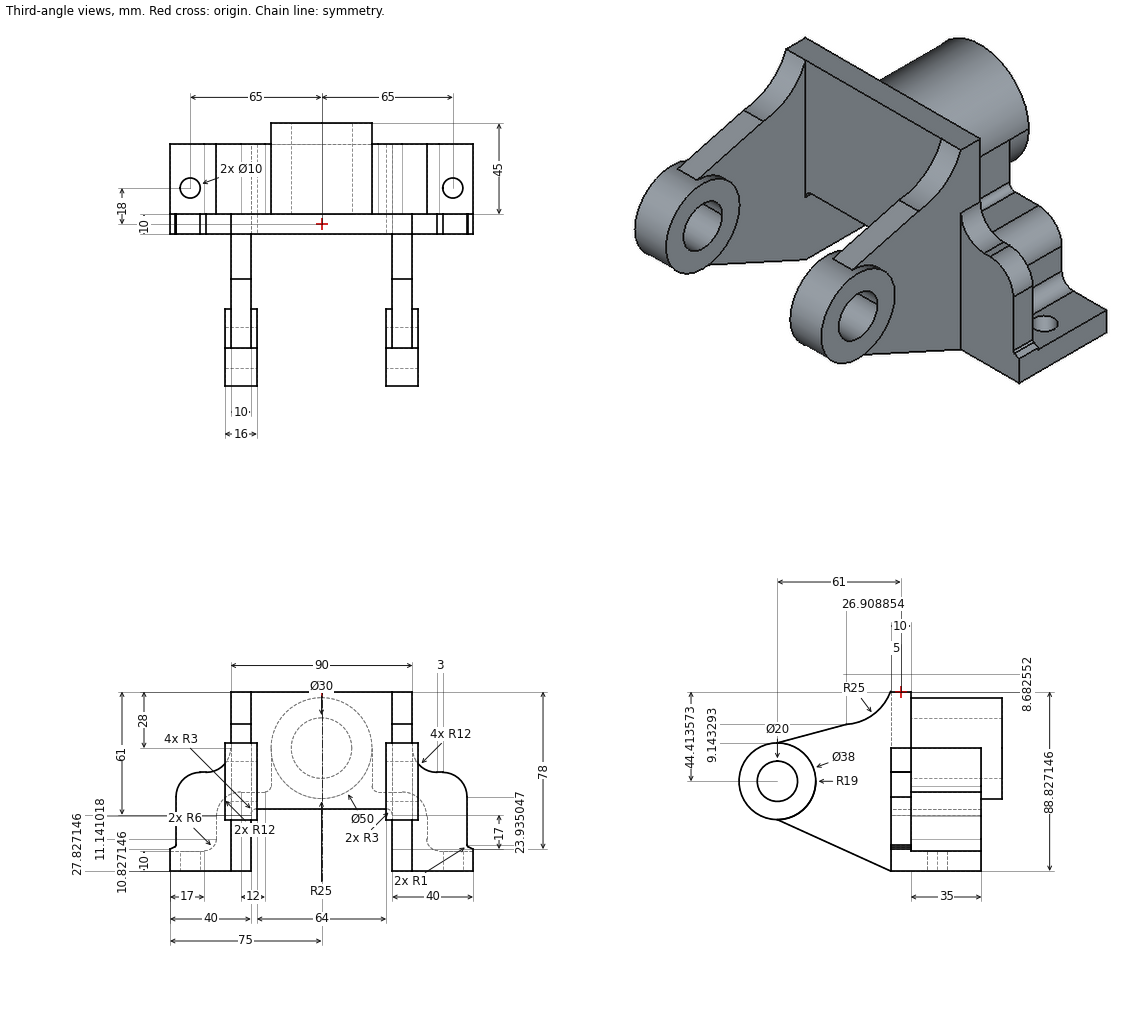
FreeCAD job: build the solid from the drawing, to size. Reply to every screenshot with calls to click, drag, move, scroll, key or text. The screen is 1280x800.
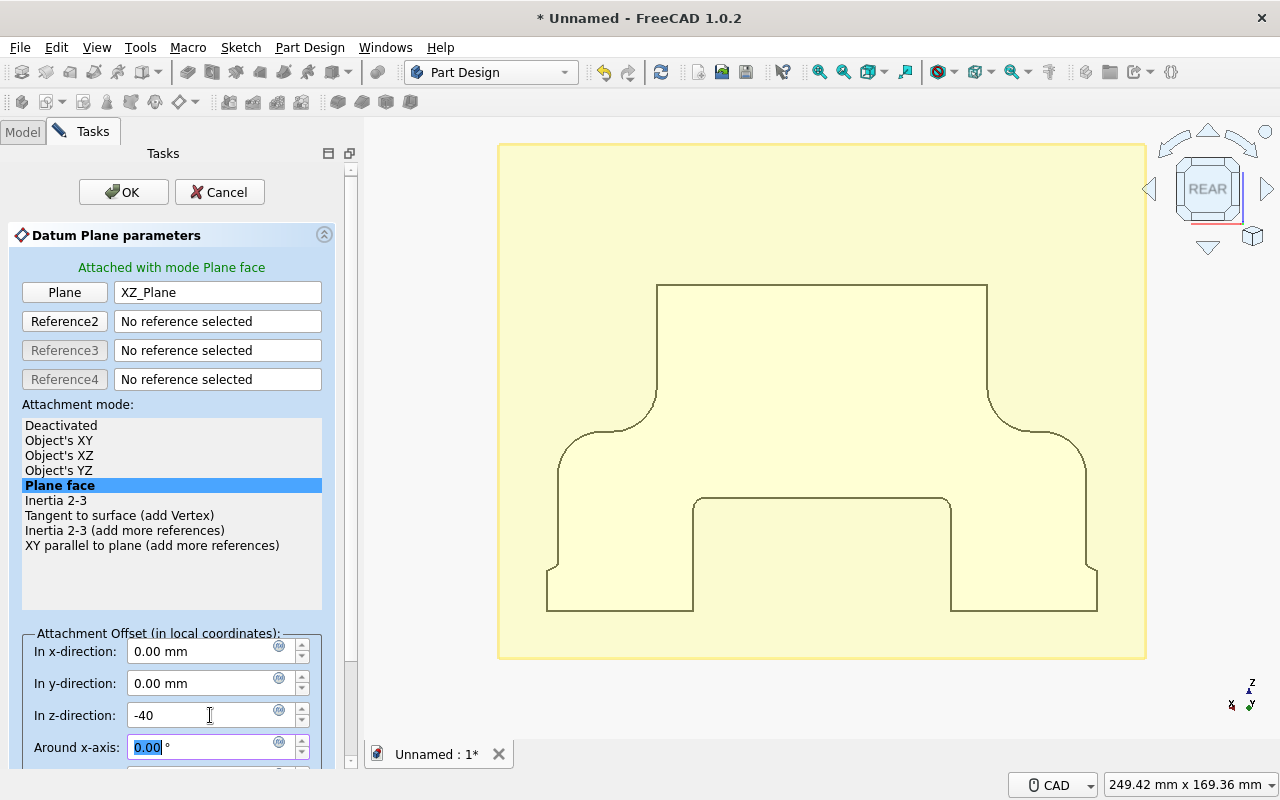
click(124, 192)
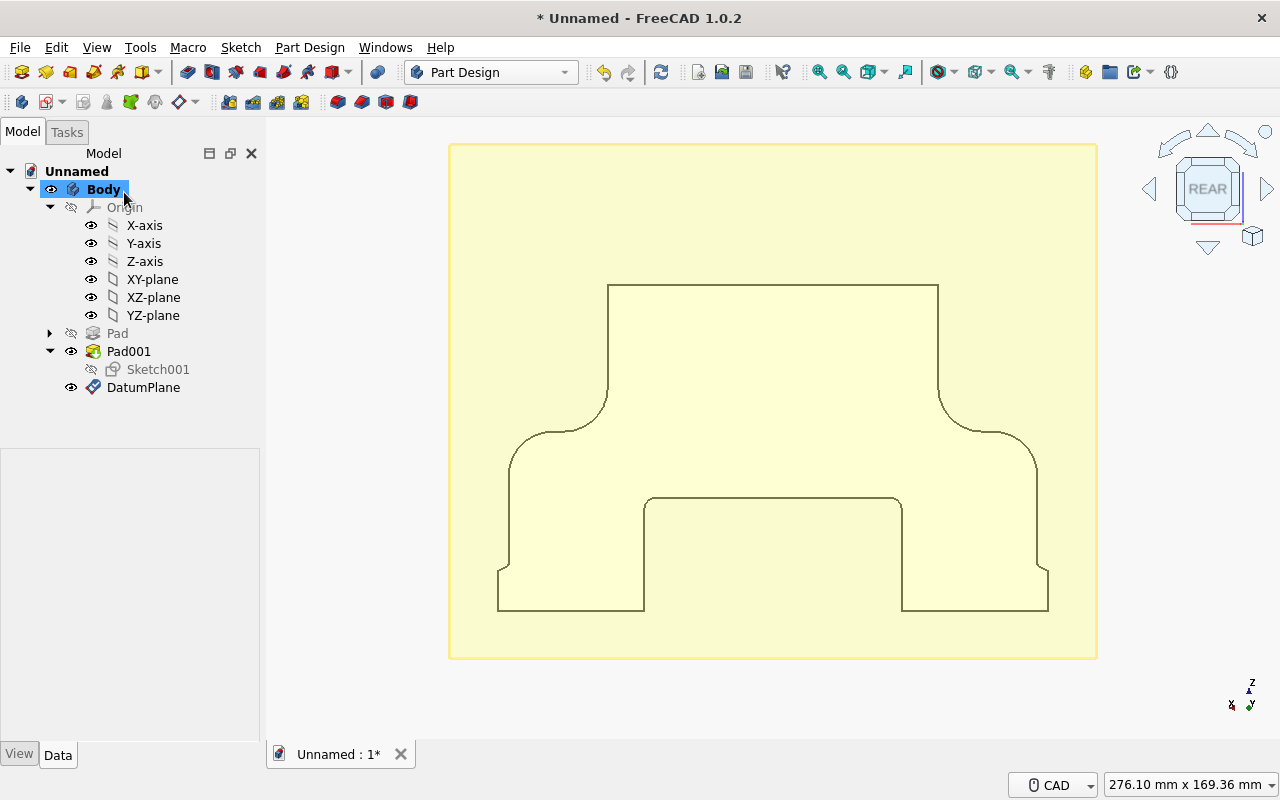
click(116, 387)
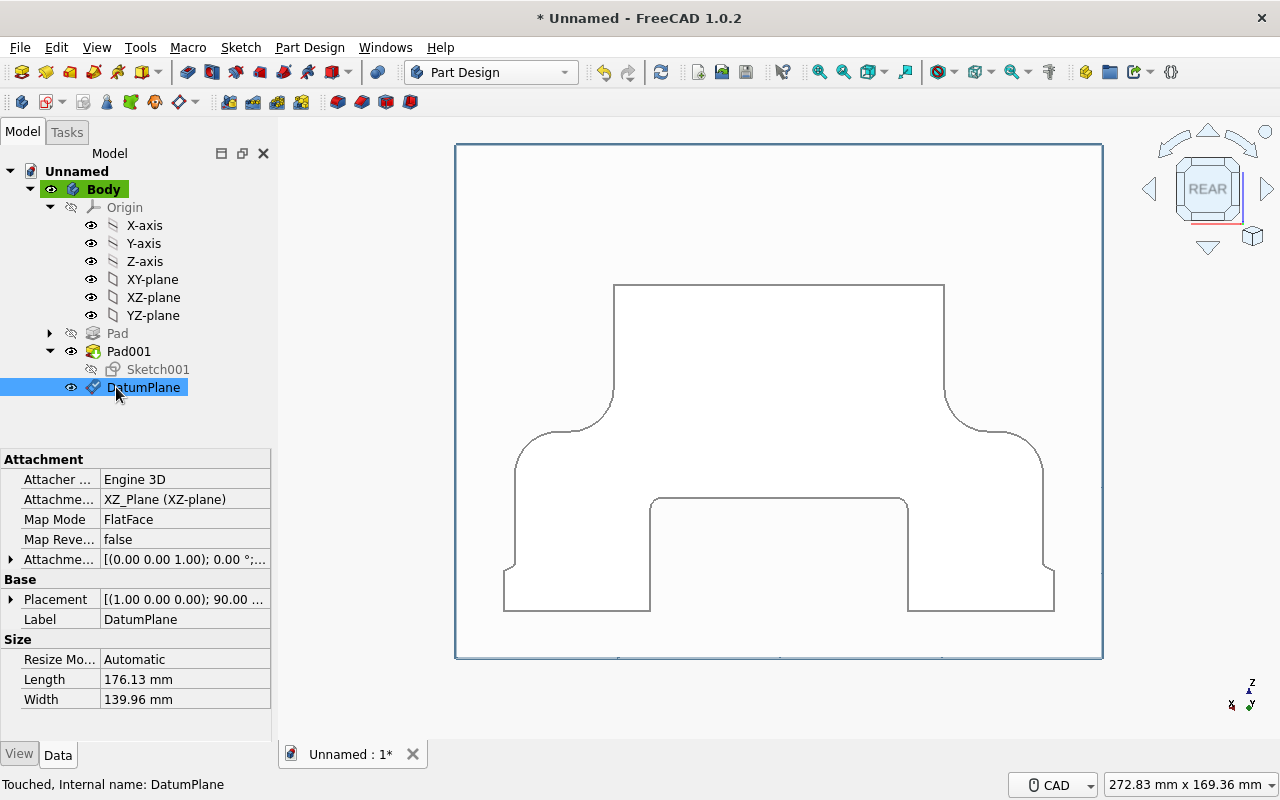
click(46, 102)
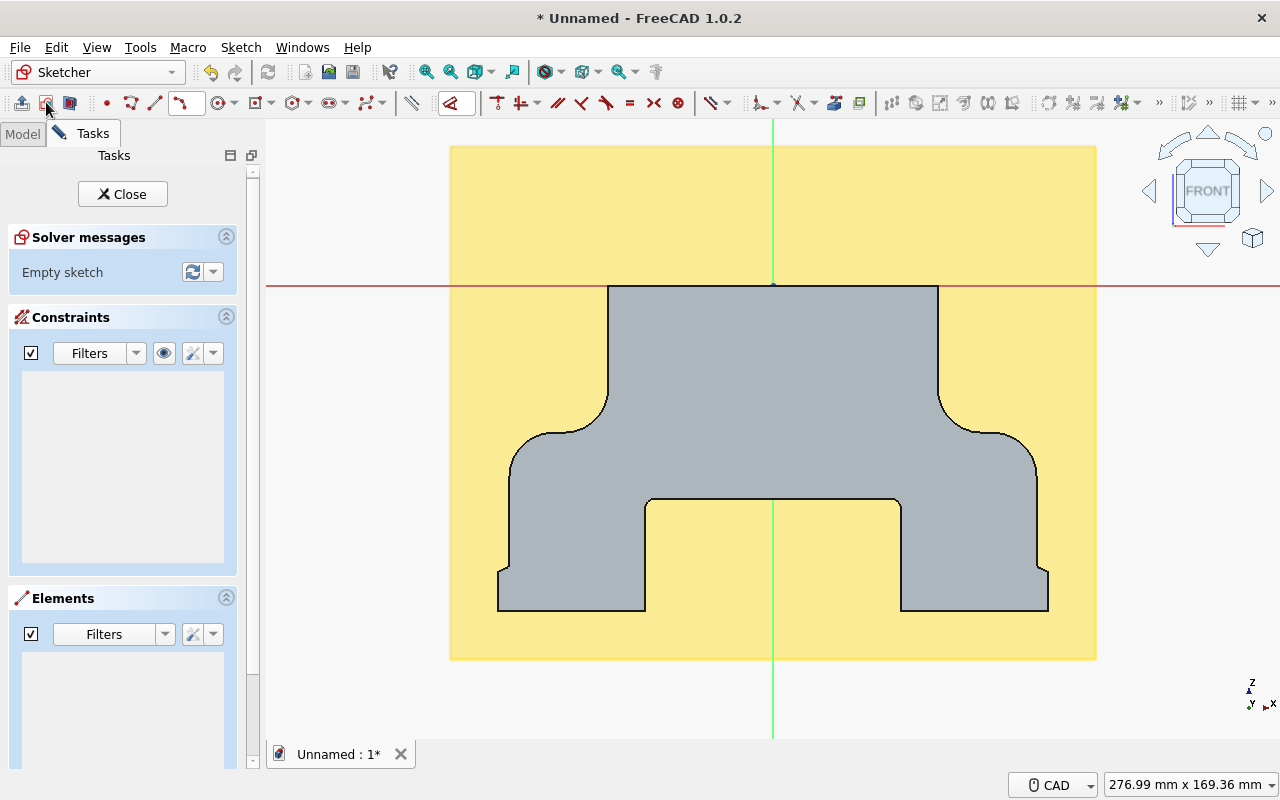
click(70, 104)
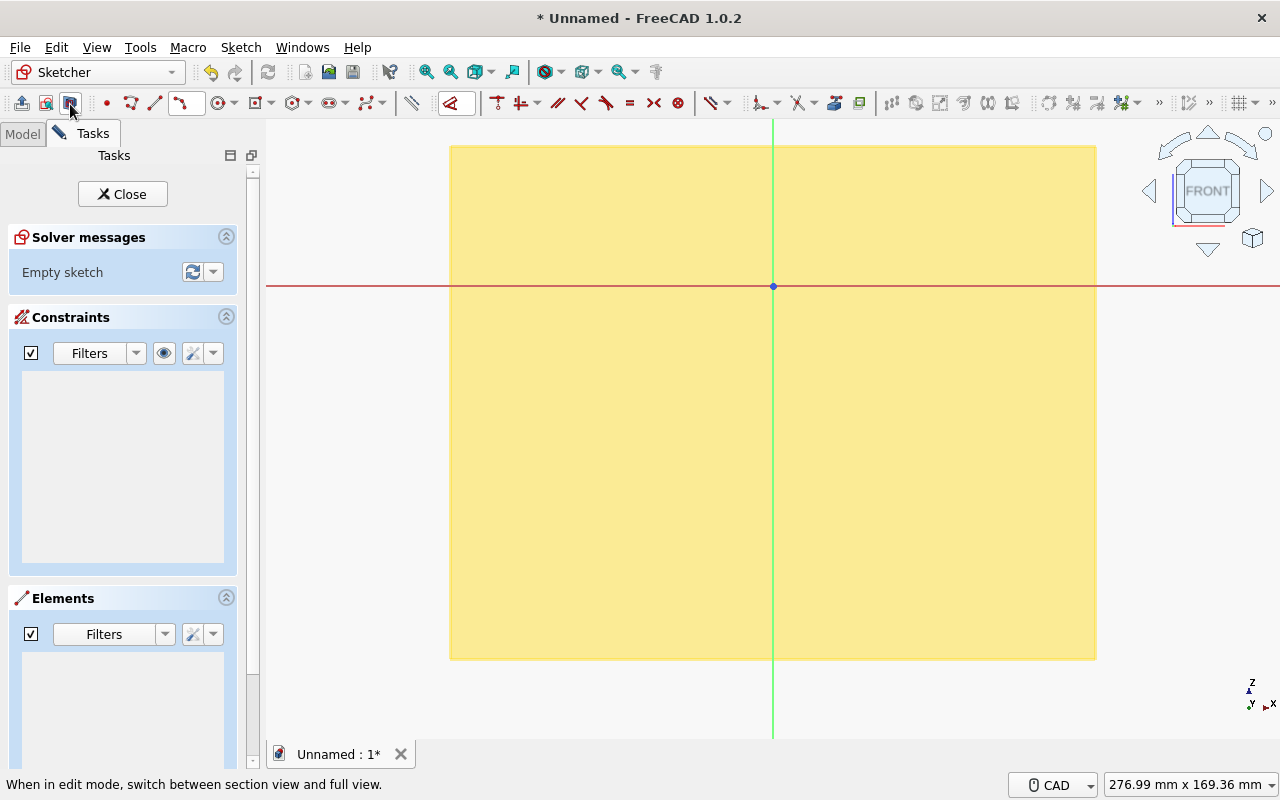
key(g)
key(m)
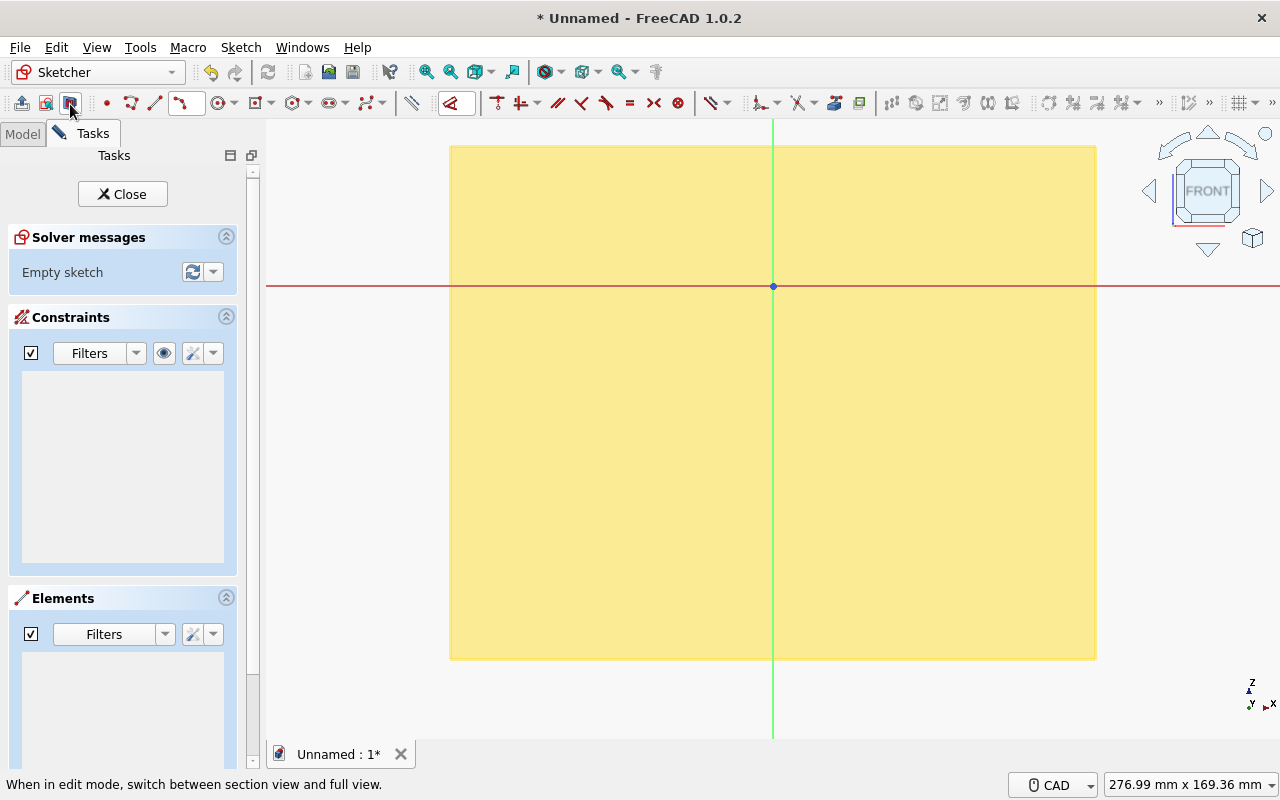
click(645, 510)
click(645, 611)
click(498, 611)
click(498, 575)
click(561, 575)
right_click(561, 575)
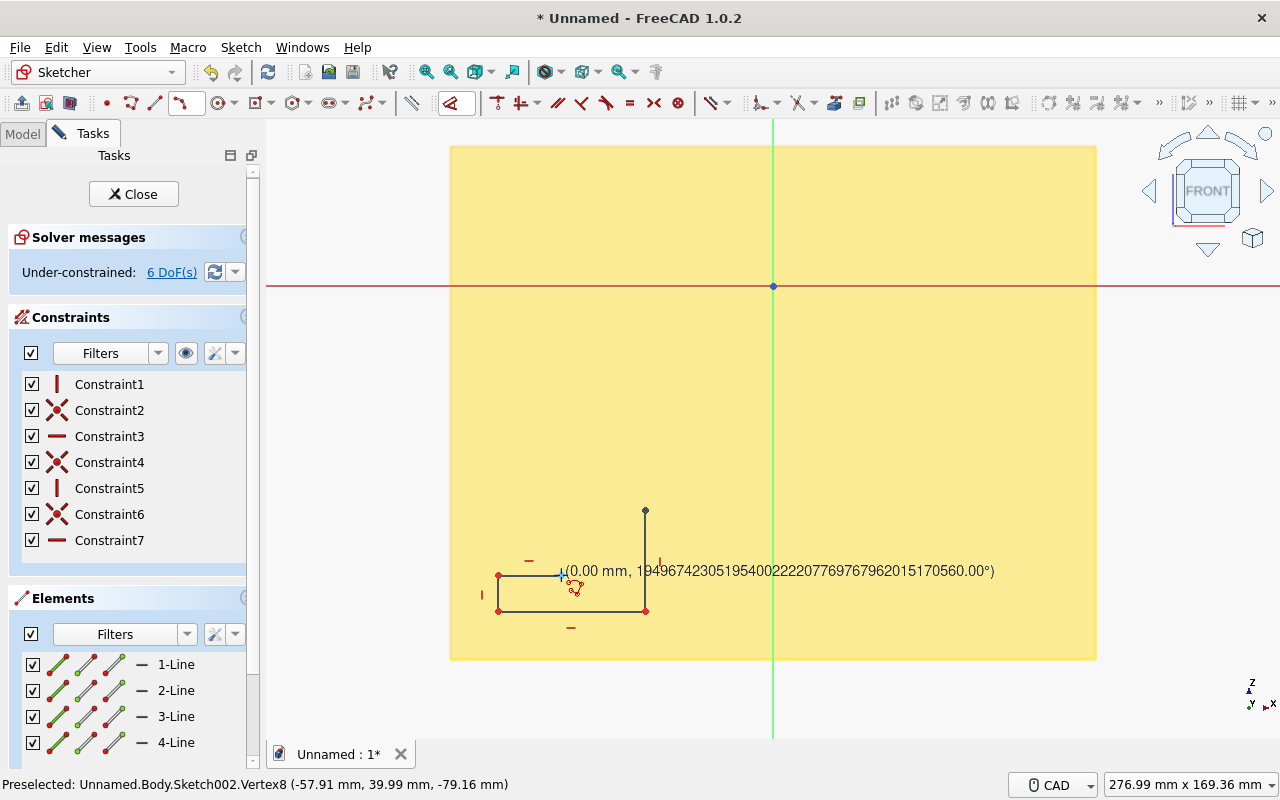
key(g)
key(l)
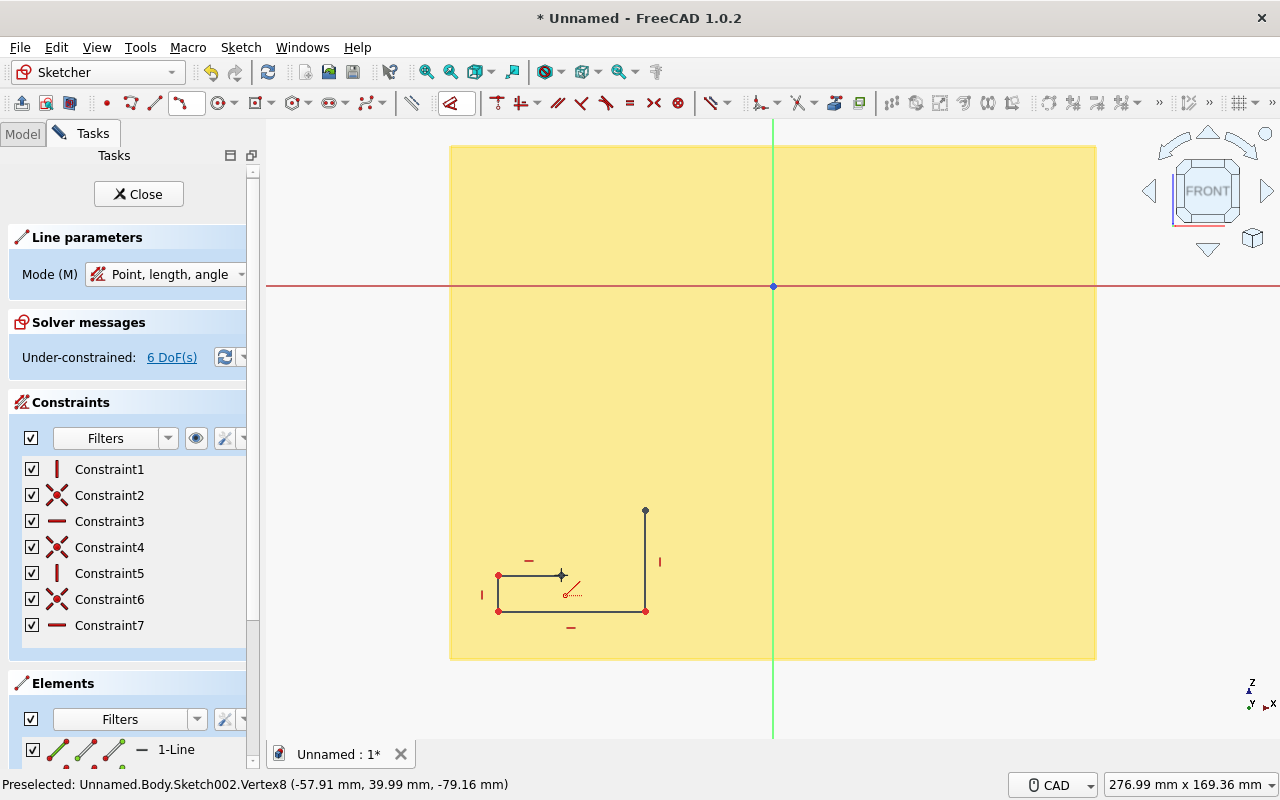
click(583, 553)
click(583, 512)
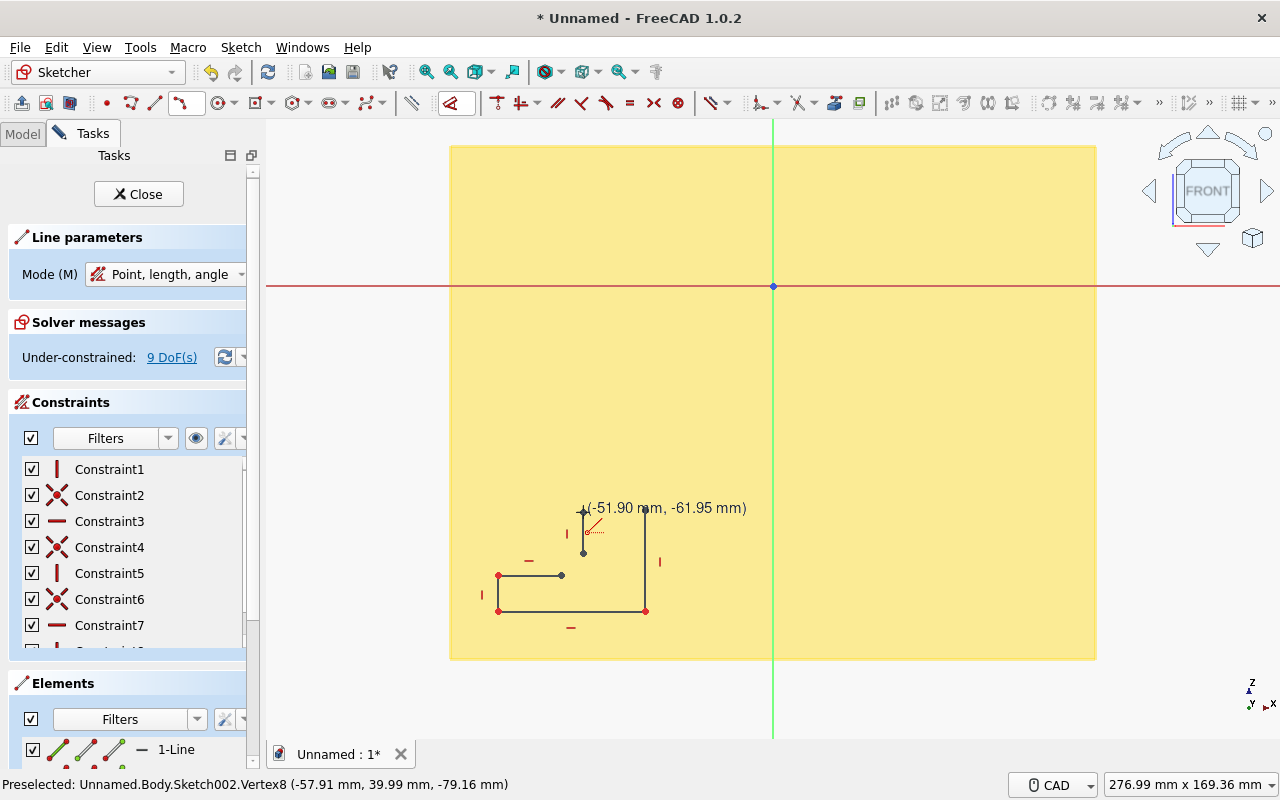
click(627, 468)
click(670, 468)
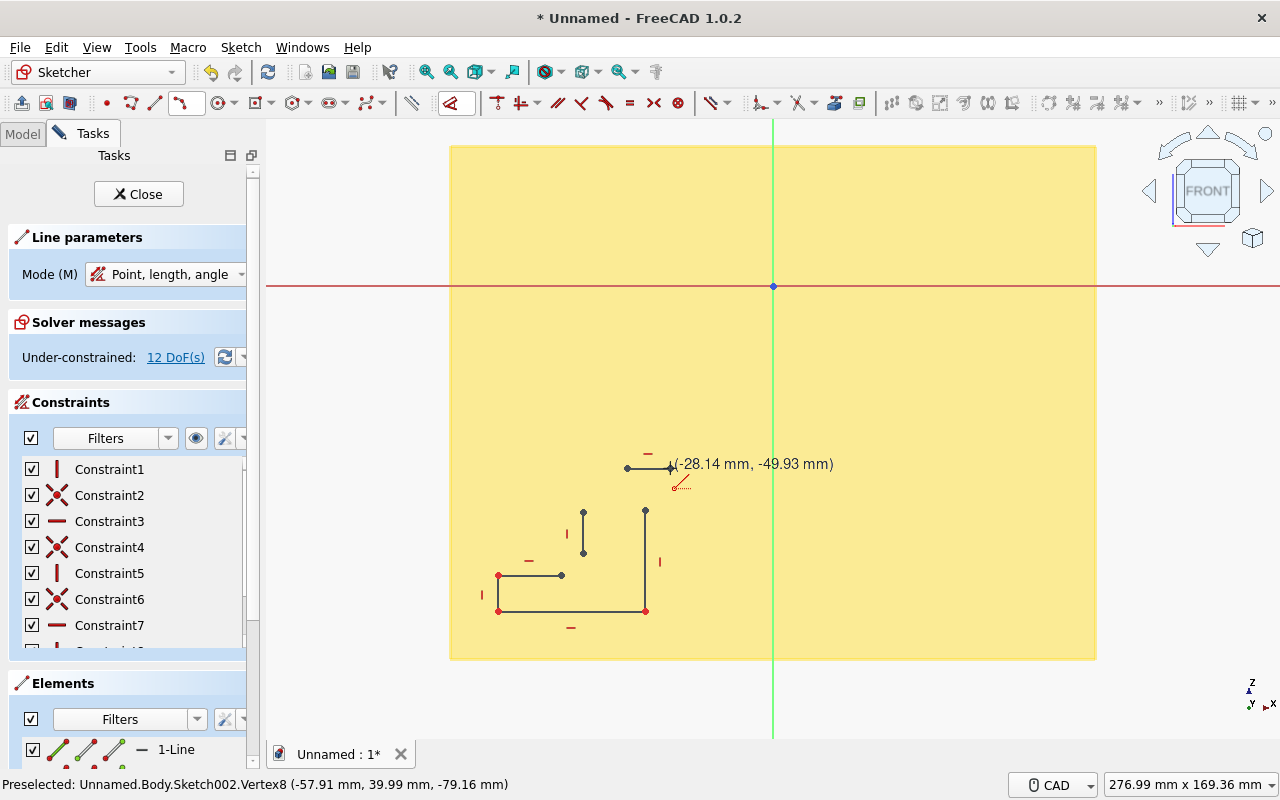
click(681, 457)
click(681, 389)